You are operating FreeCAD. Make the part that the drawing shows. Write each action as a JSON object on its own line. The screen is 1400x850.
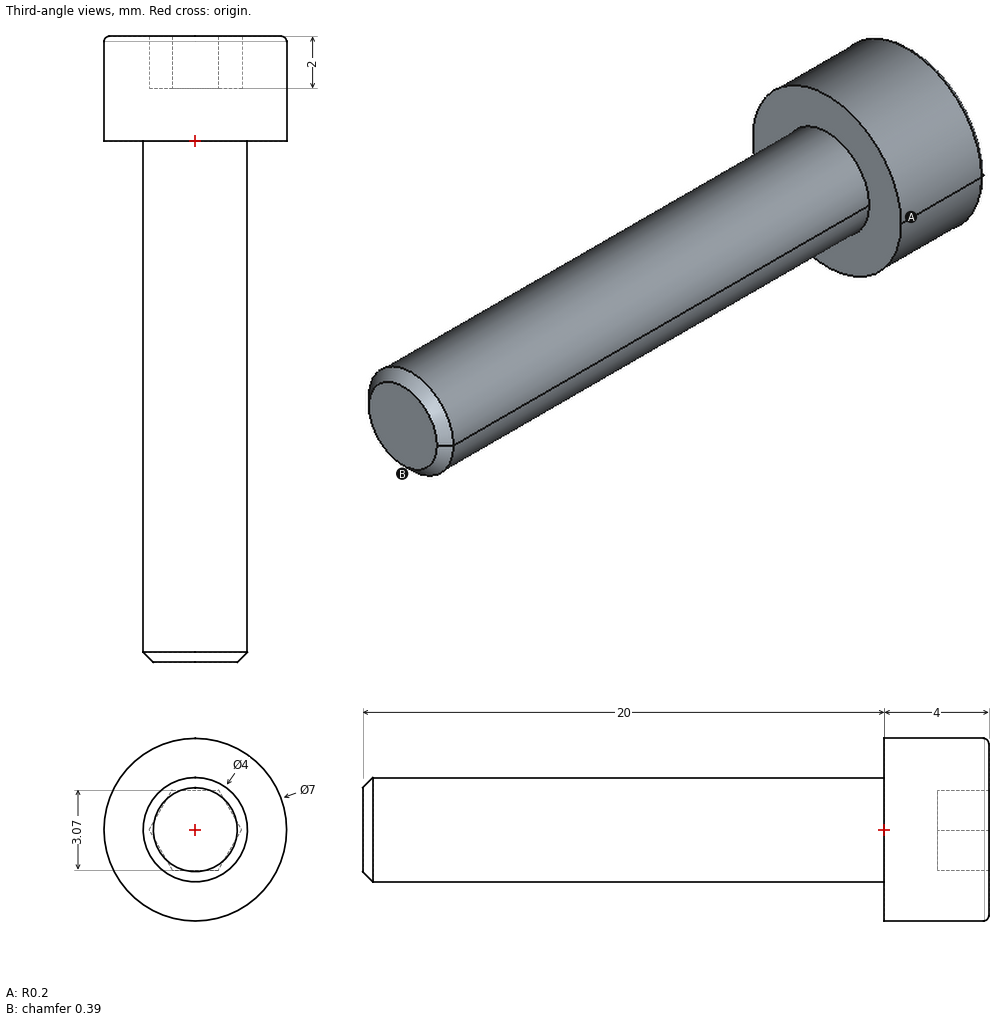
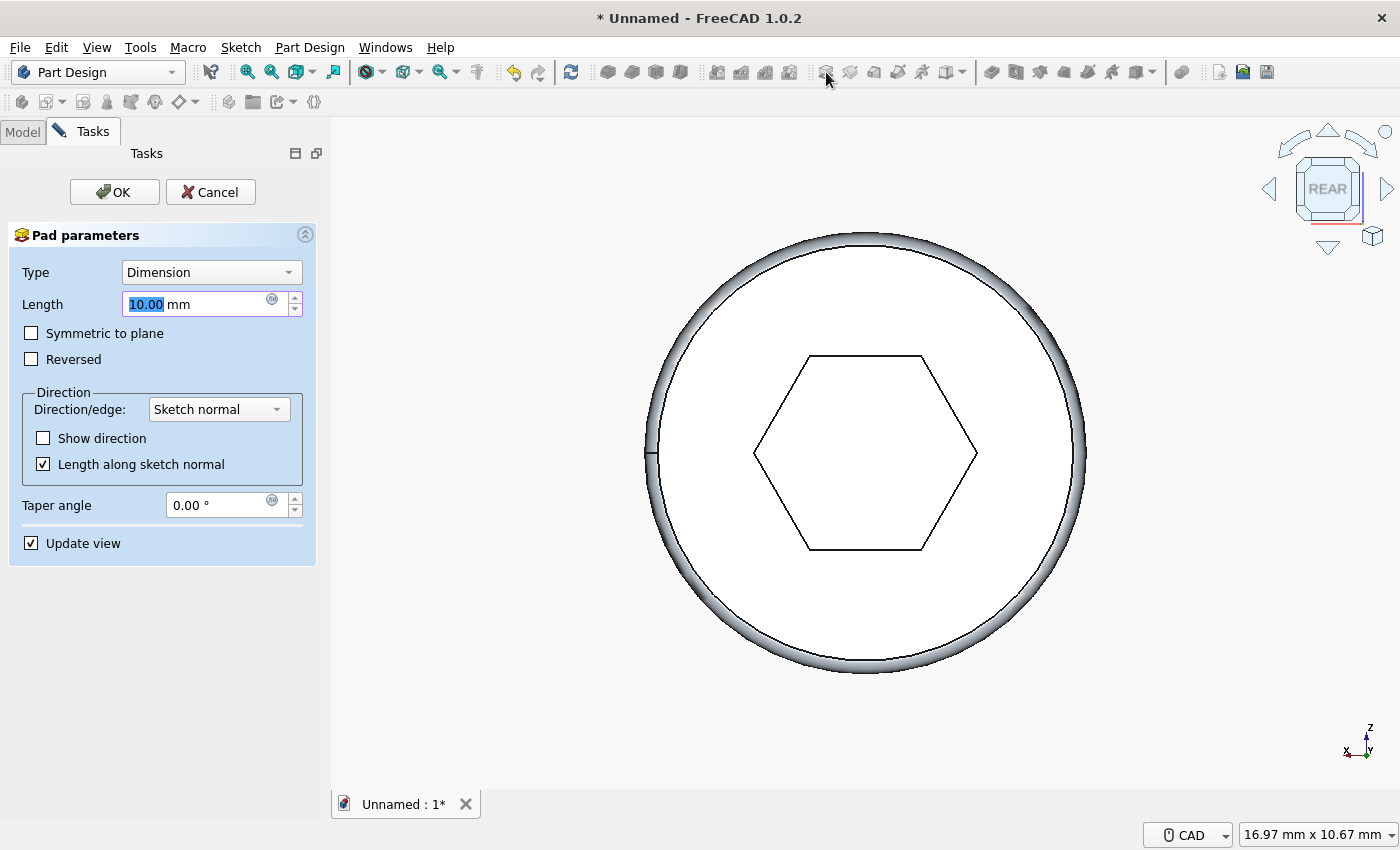
{"action": "type", "text": "20"}
{"action": "key", "text": "Tab"}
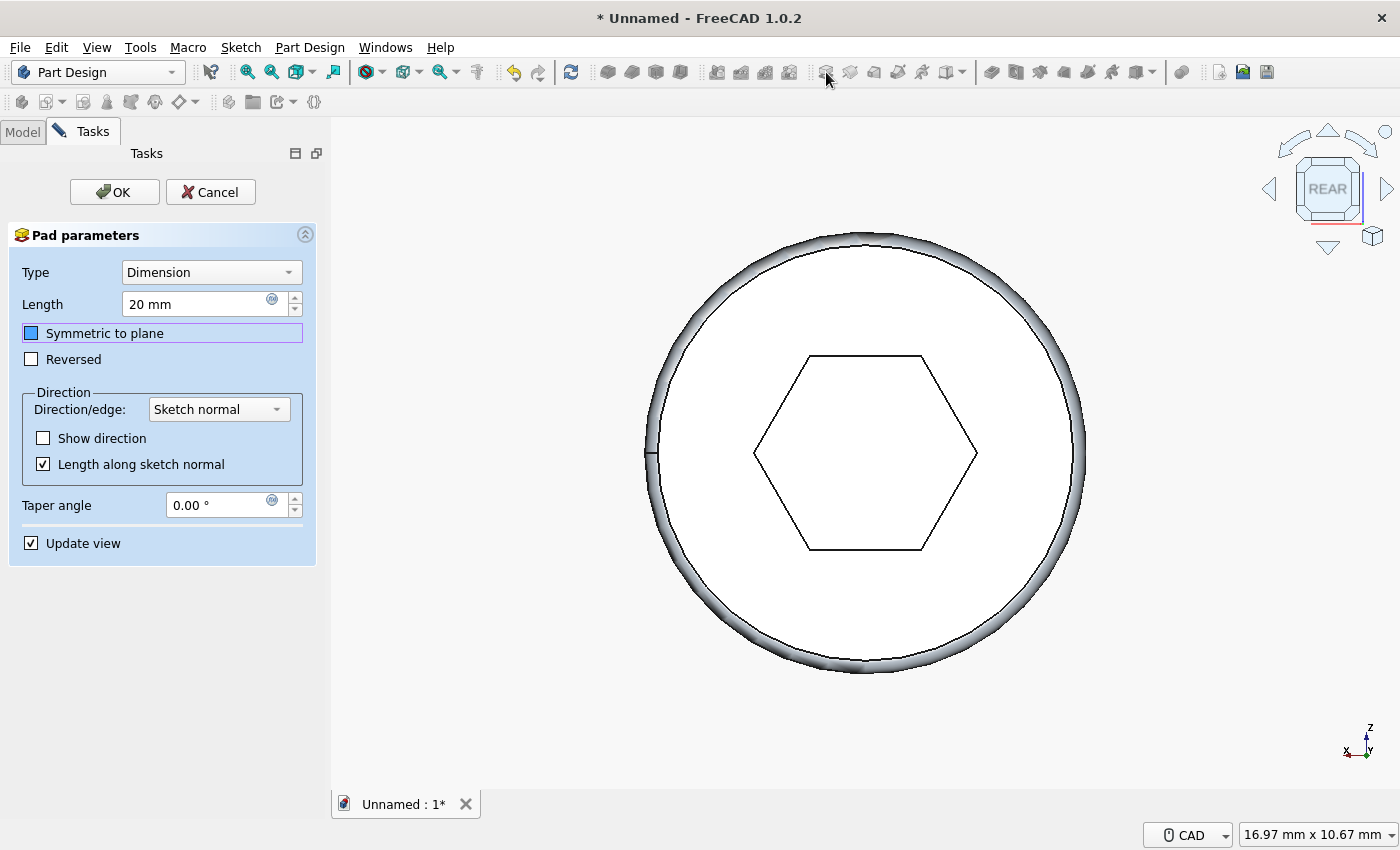
{"action": "left_click", "coordinate": [115, 192]}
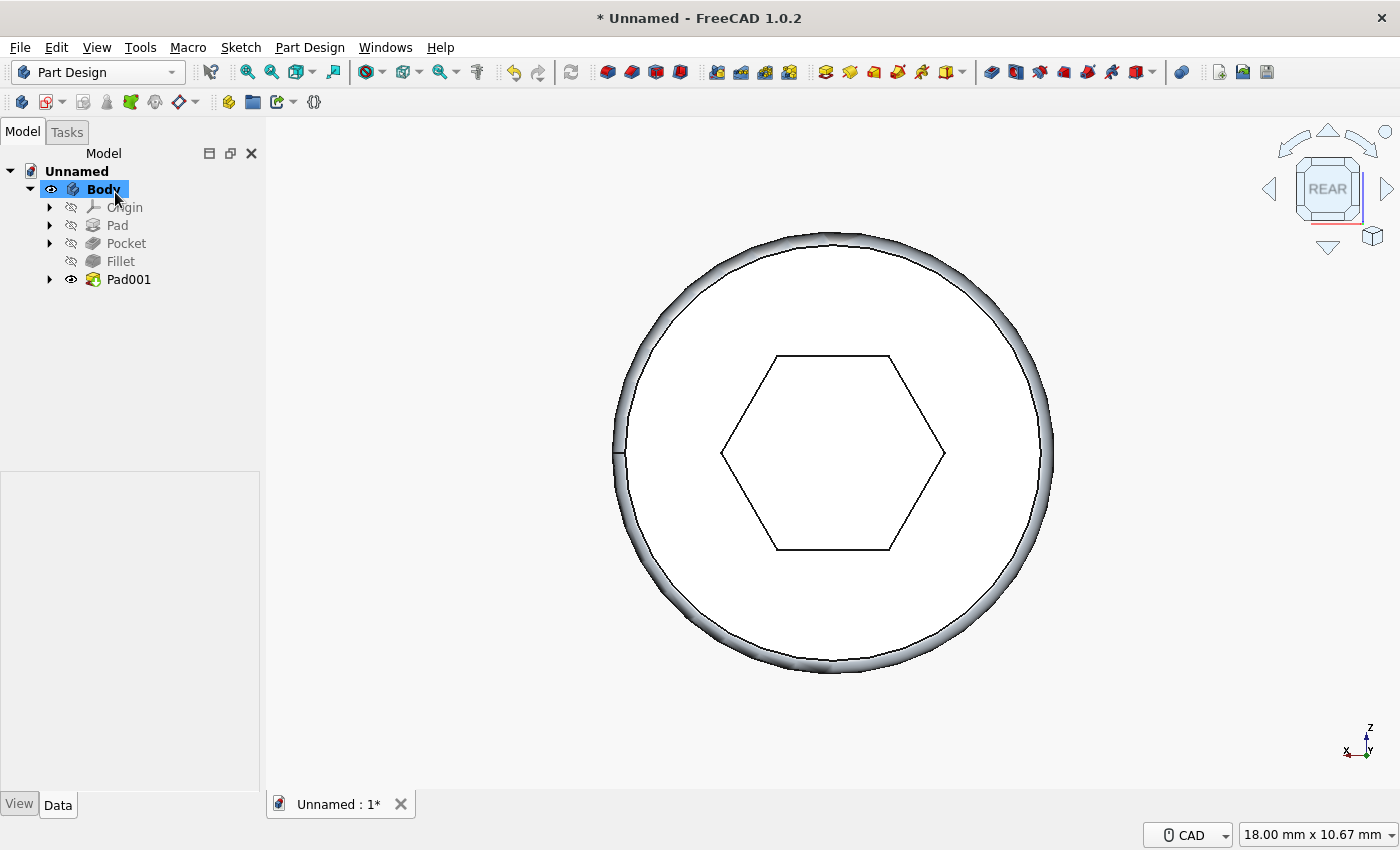
{"action": "key", "text": "0"}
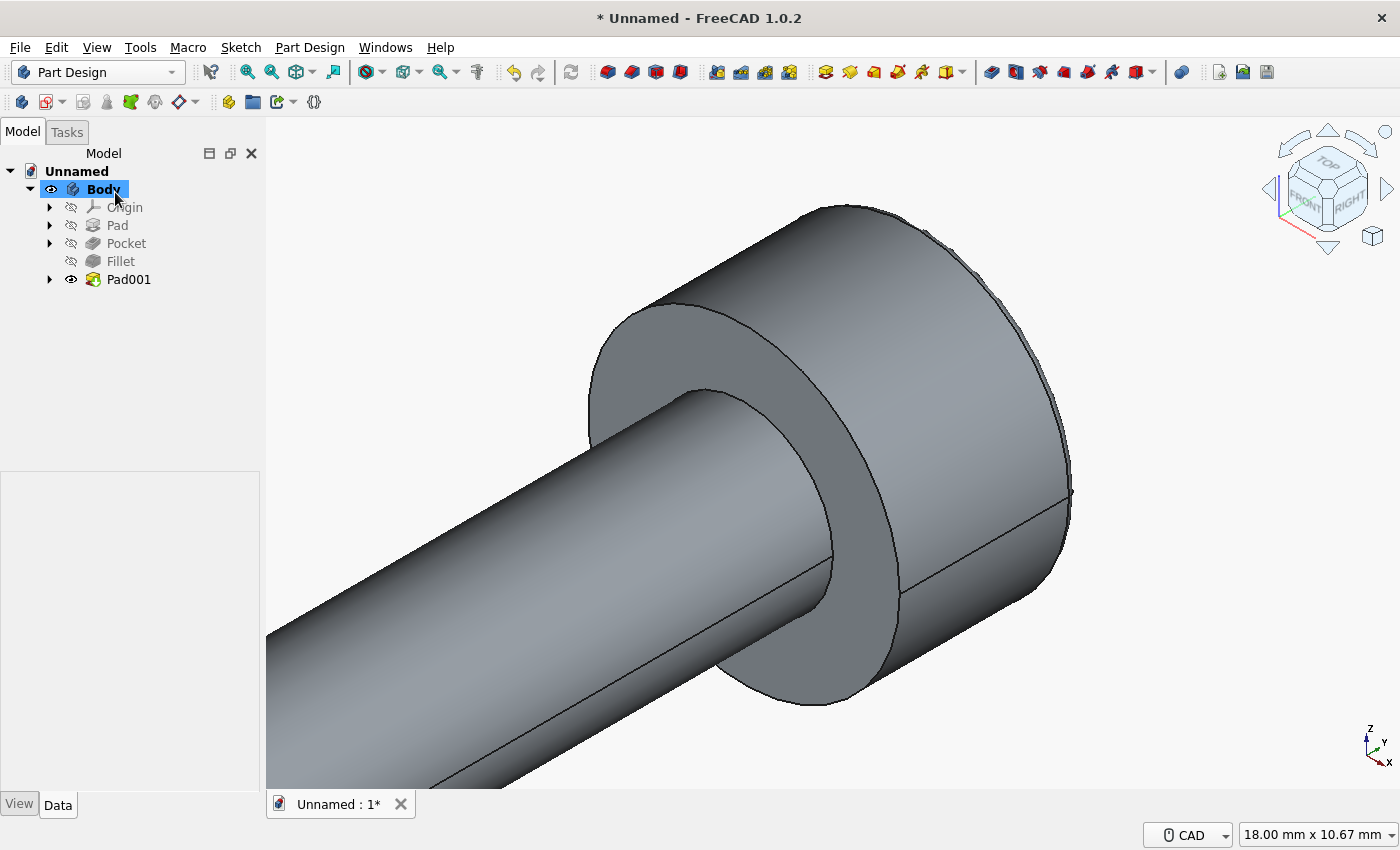
{"action": "key", "text": "v f"}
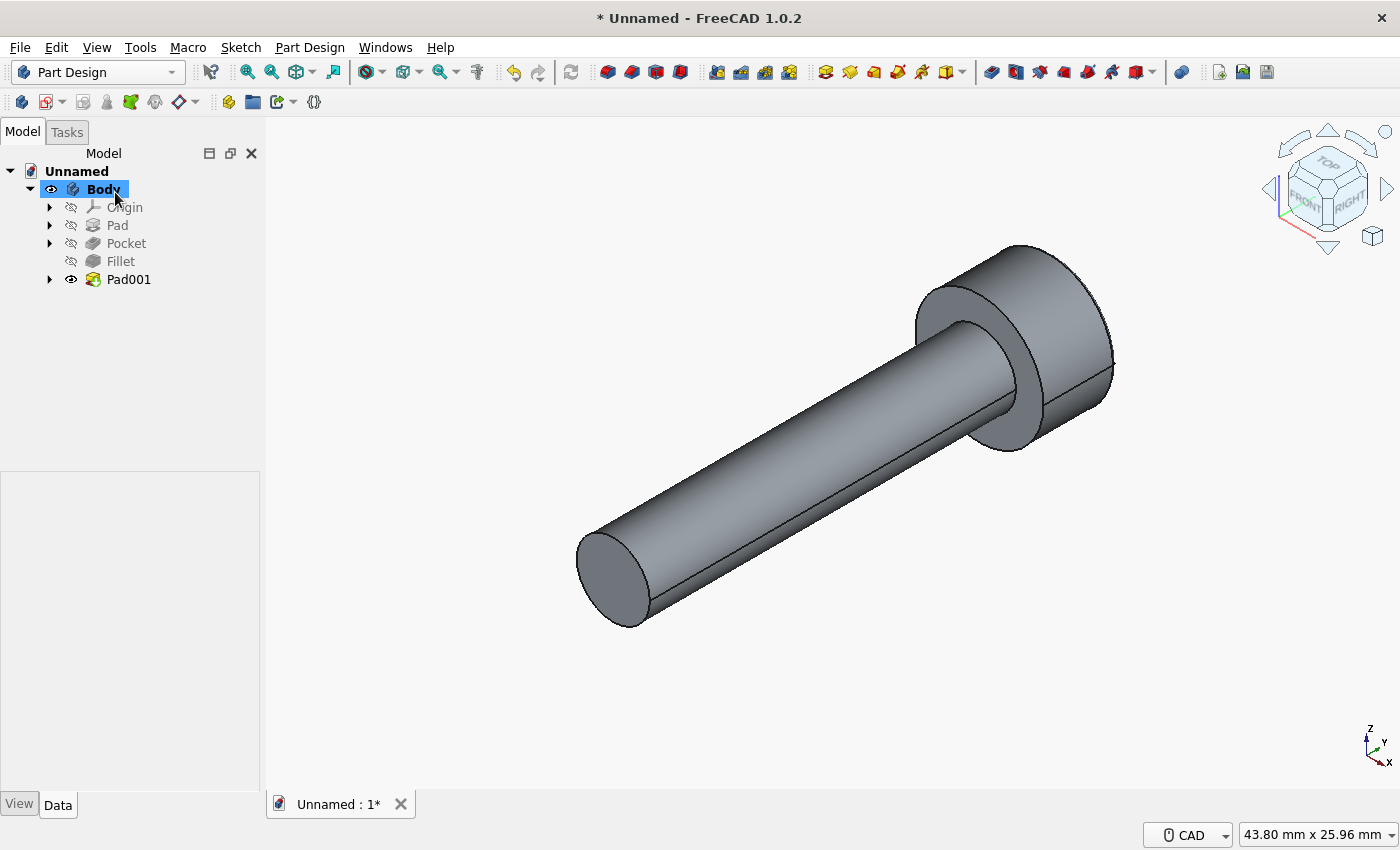
{"action": "left_click", "coordinate": [584, 537]}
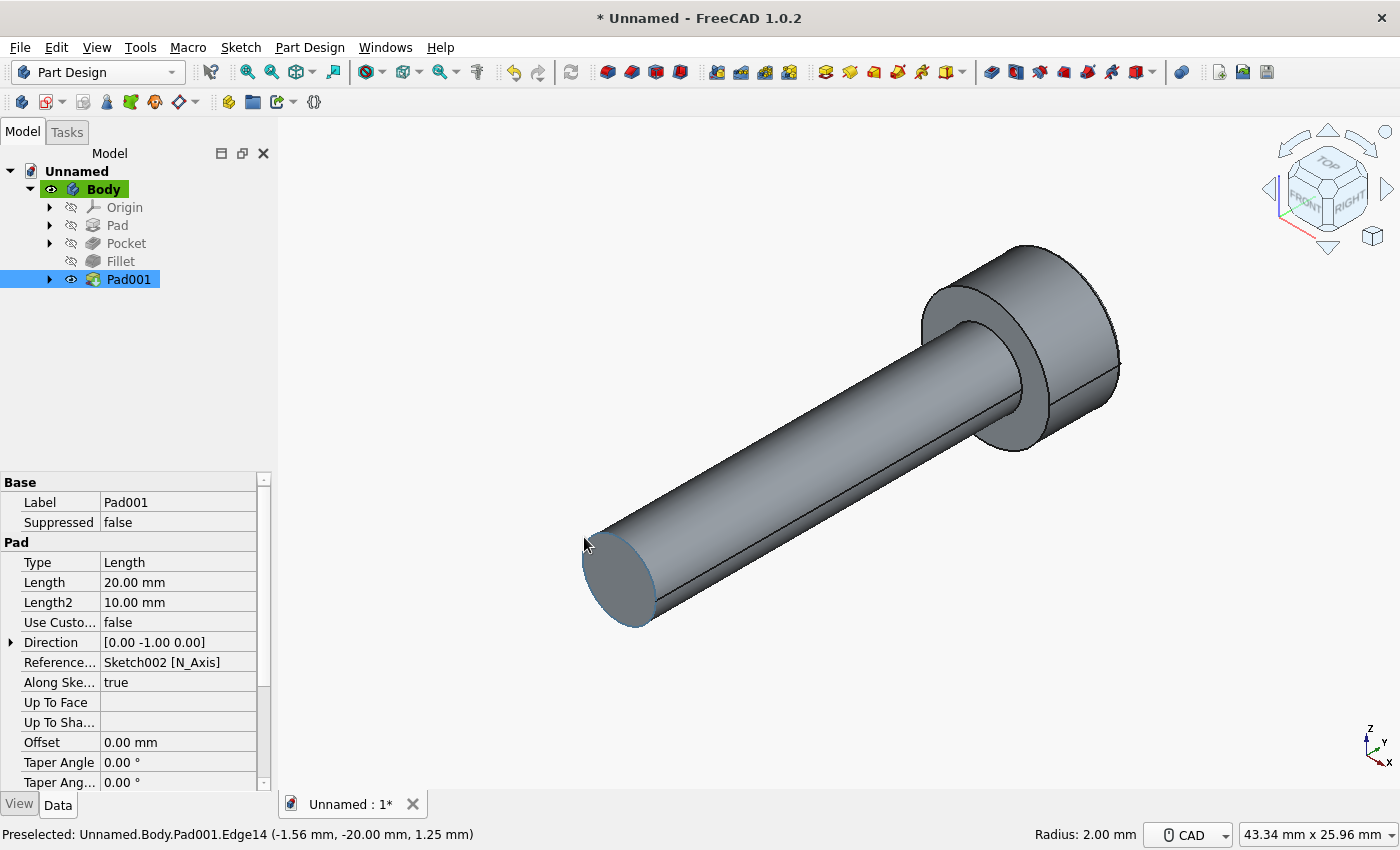
{"action": "left_click", "coordinate": [632, 72]}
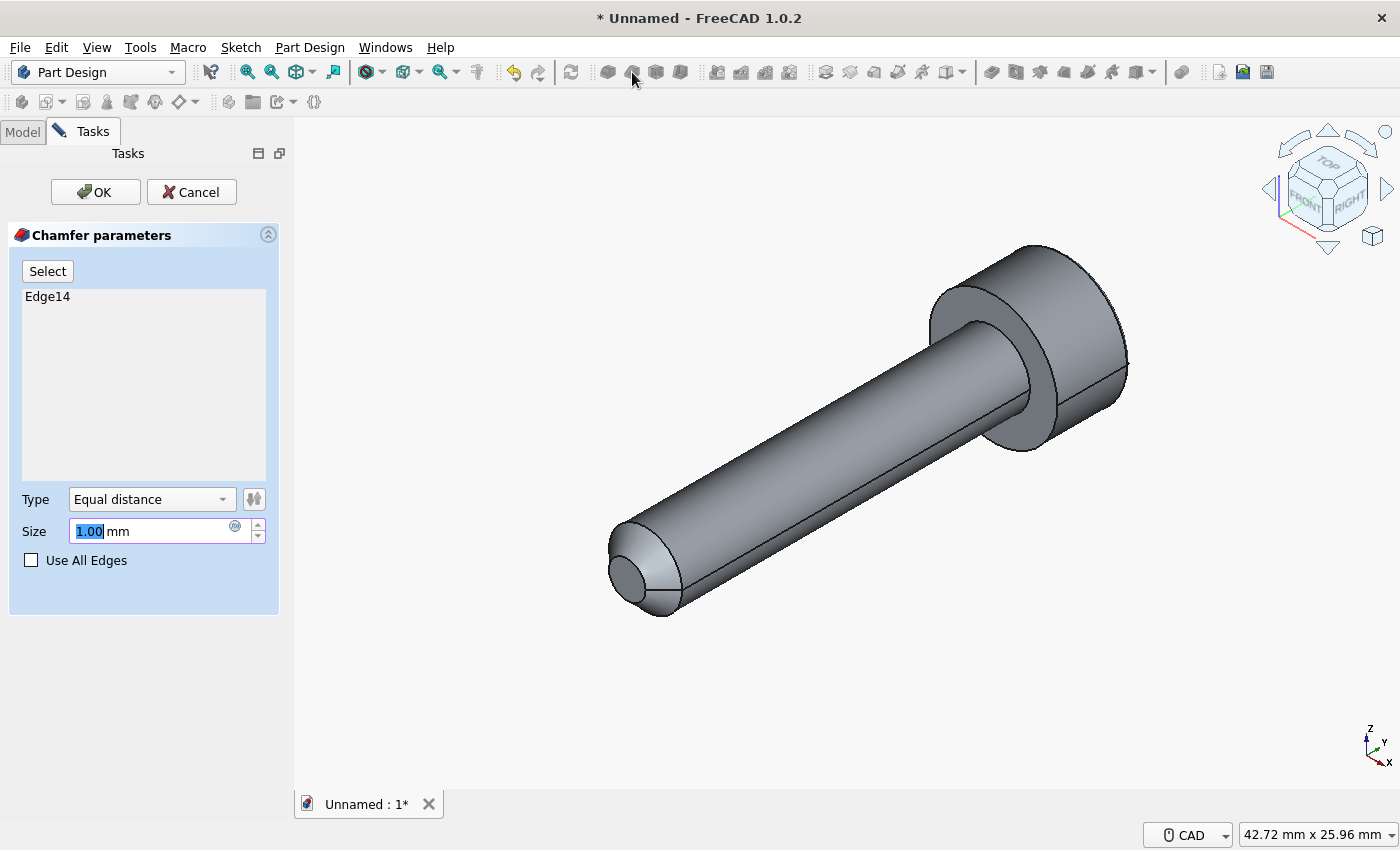
{"action": "type", "text": "0.39"}
{"action": "key", "text": "Tab"}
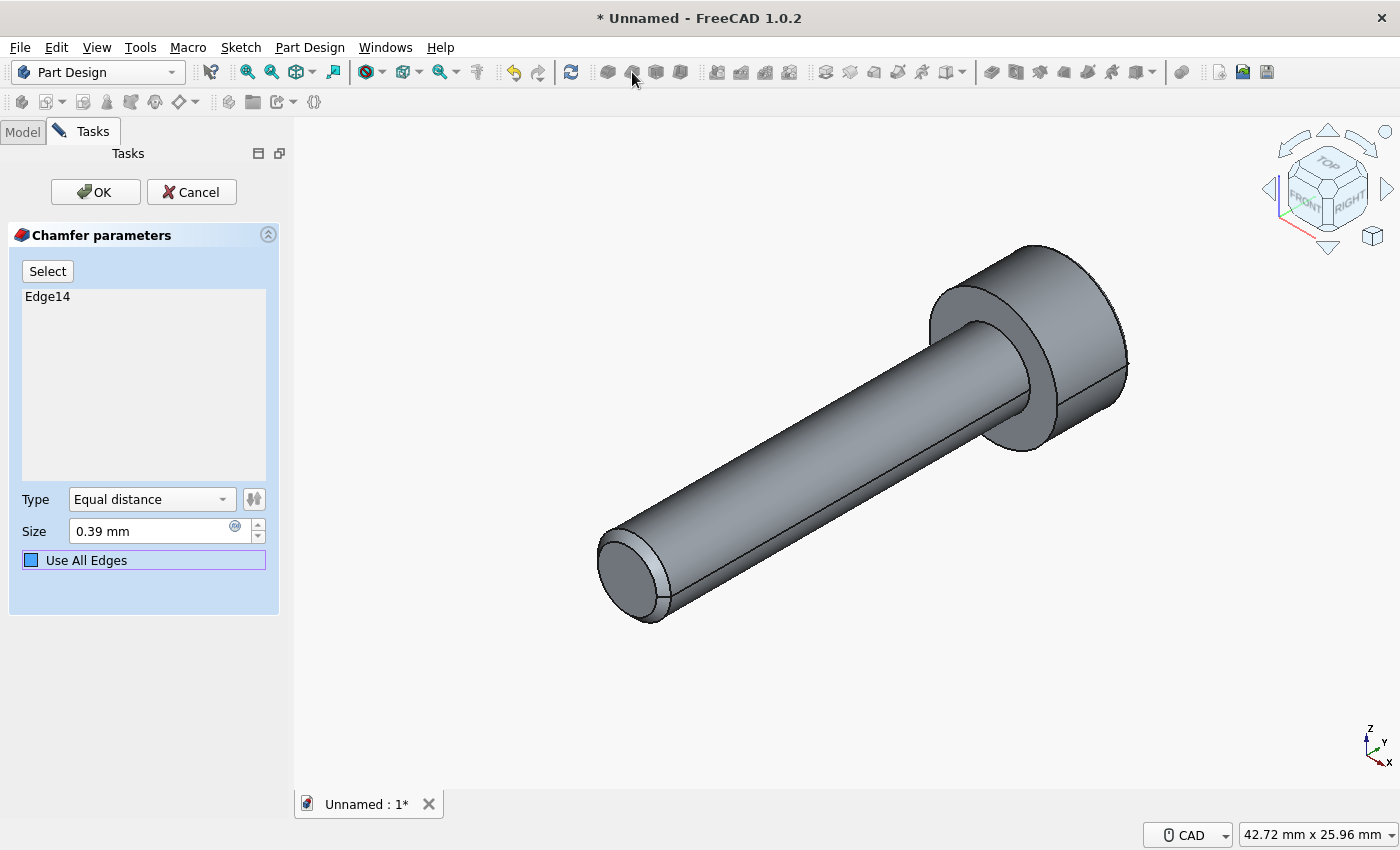
{"action": "left_click", "coordinate": [96, 192]}